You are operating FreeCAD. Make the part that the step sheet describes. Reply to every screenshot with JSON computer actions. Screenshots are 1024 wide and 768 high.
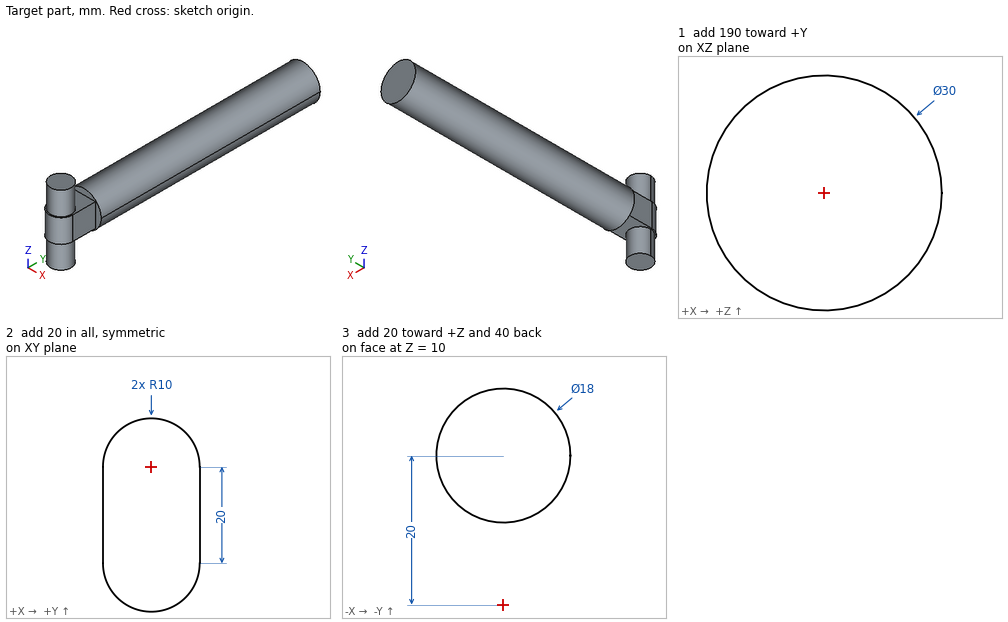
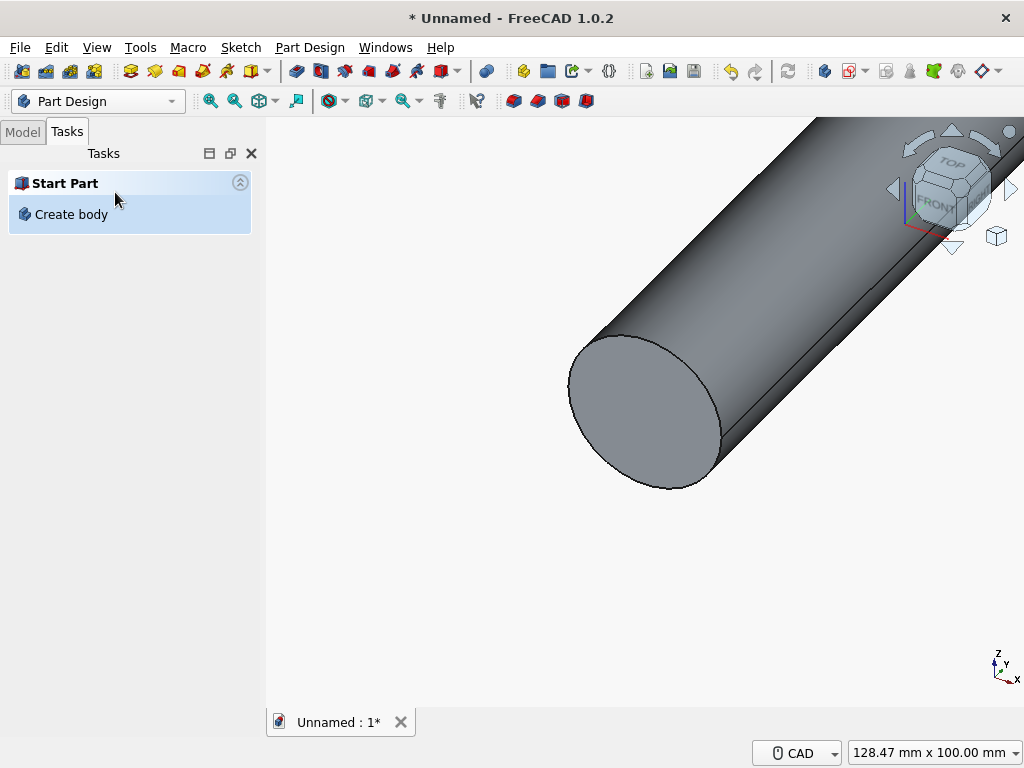
{"action": "left_click", "coordinate": [212, 102]}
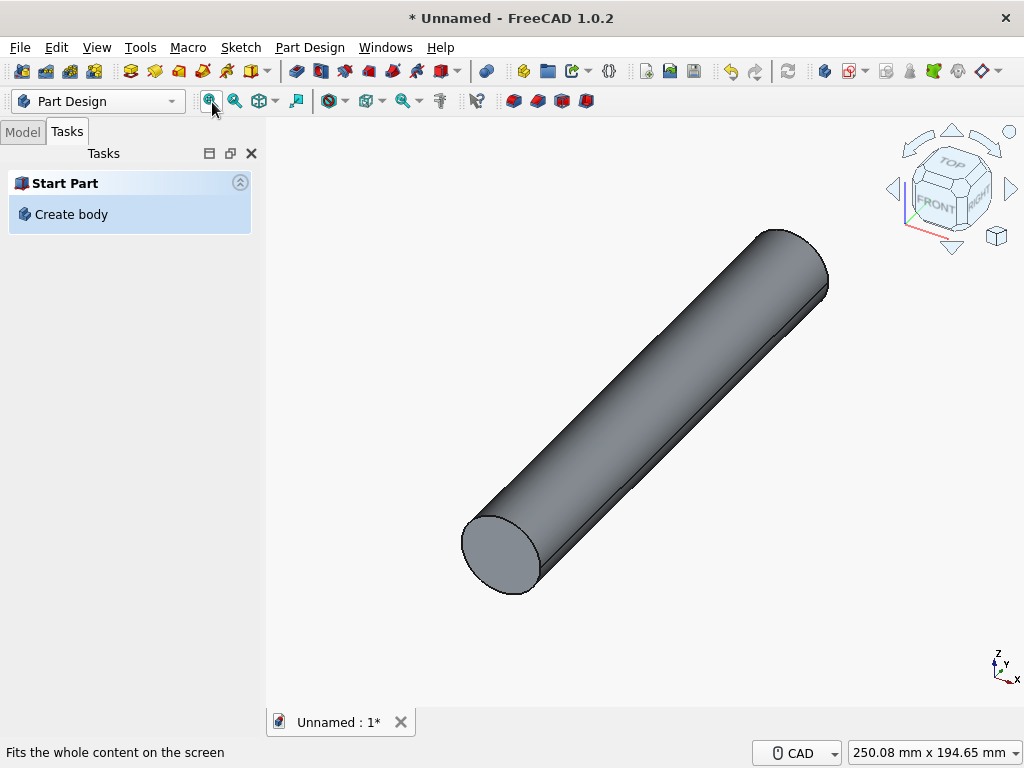
{"action": "left_click", "coordinate": [850, 72]}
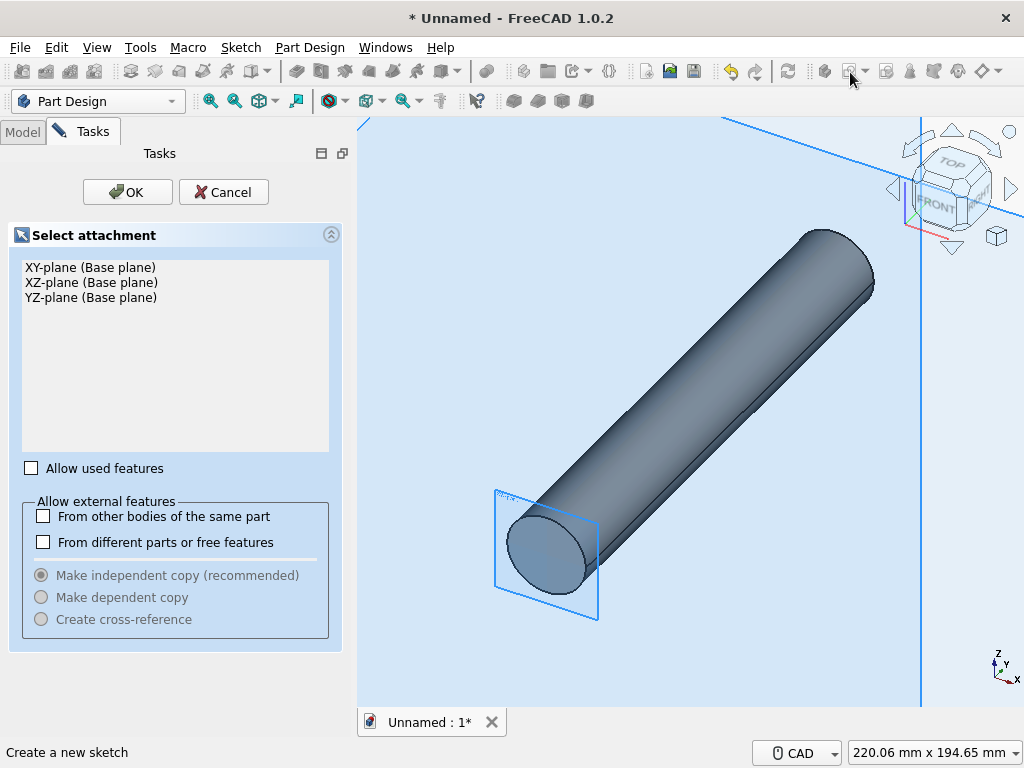
{"action": "left_click", "coordinate": [82, 268]}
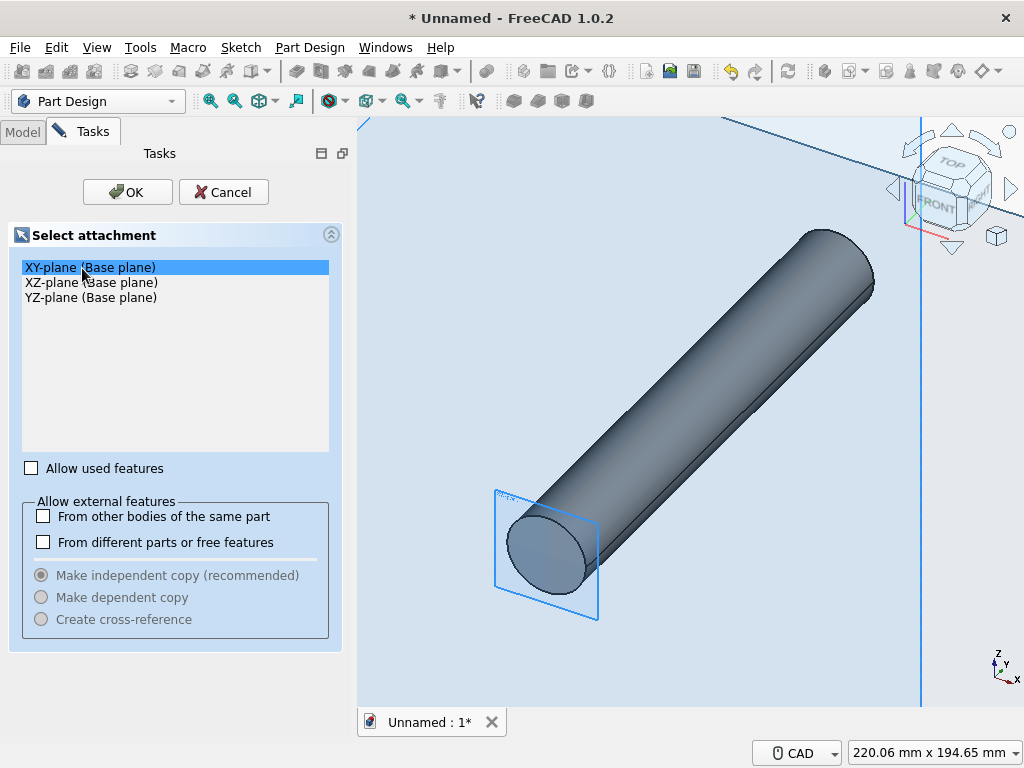
{"action": "left_click", "coordinate": [128, 192]}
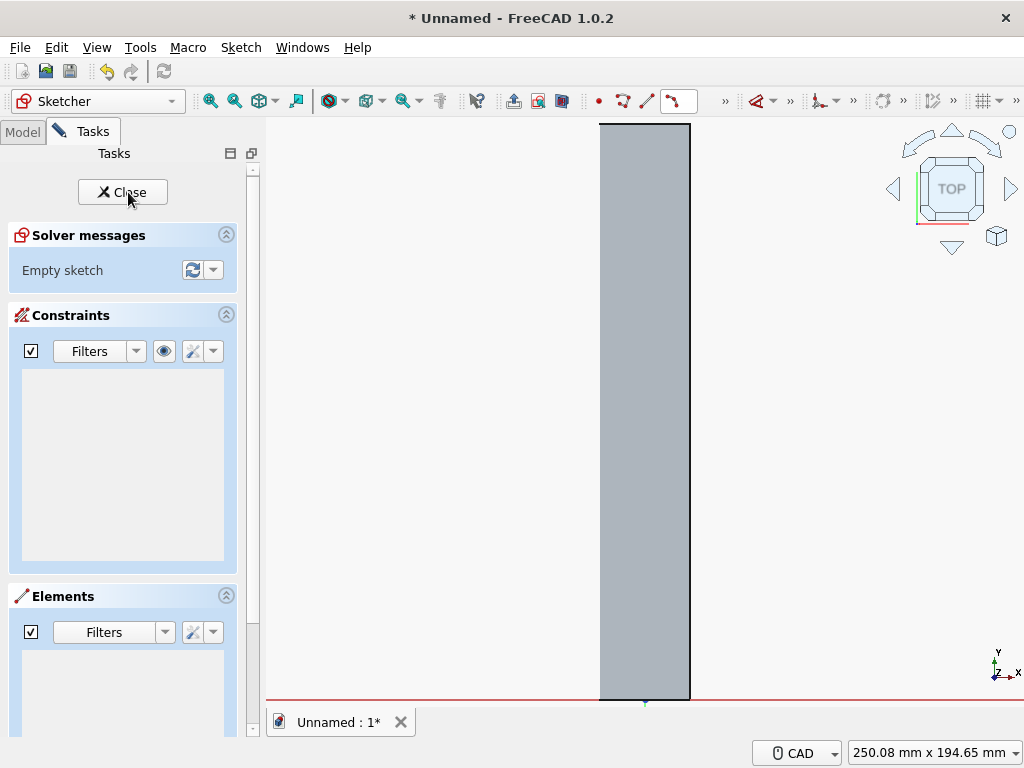
{"action": "key", "text": "q s"}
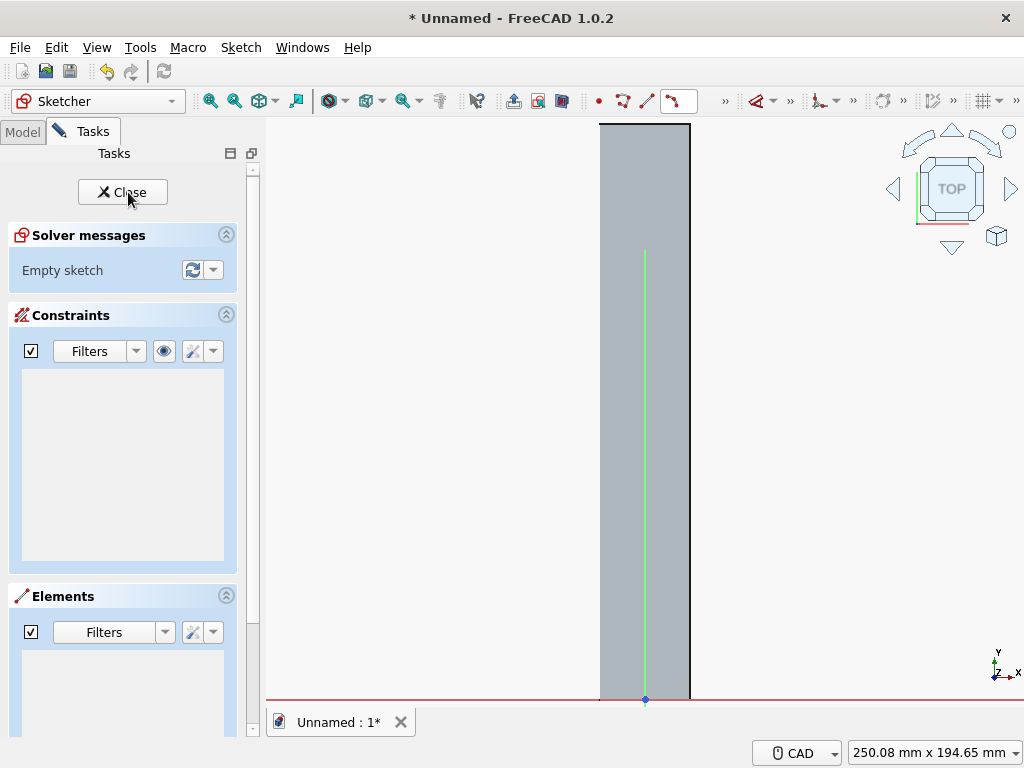
{"action": "scroll", "coordinate": [576, 412], "scroll_direction": "down", "scroll_amount": 5}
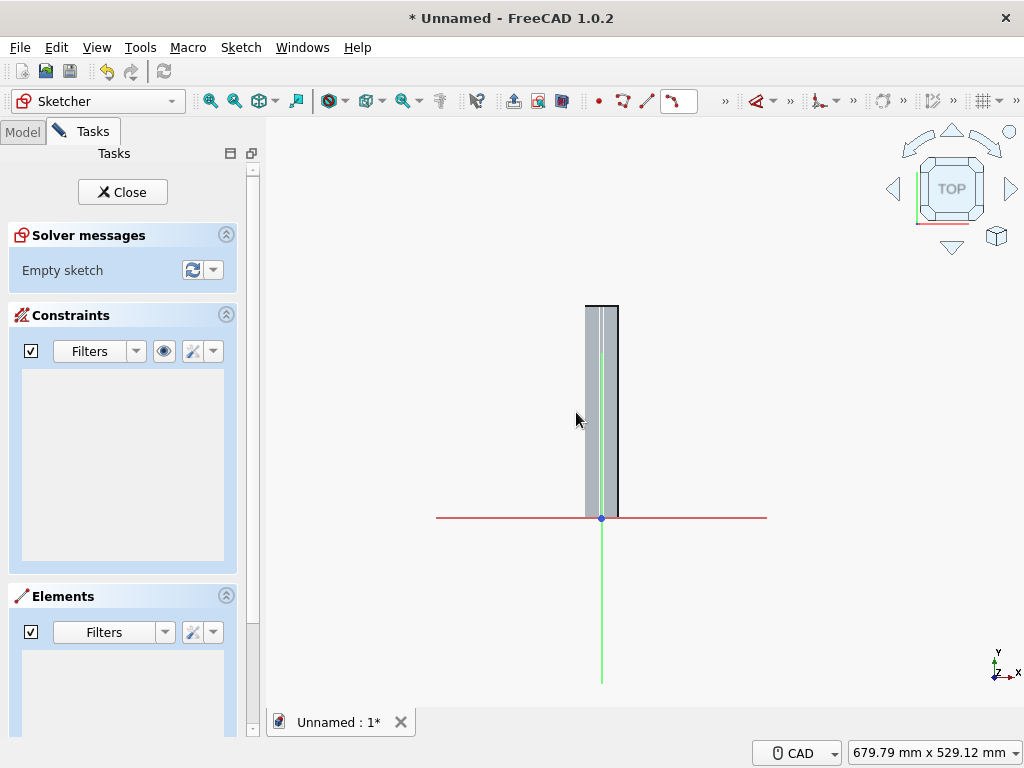
{"action": "scroll", "coordinate": [605, 544], "scroll_direction": "up", "scroll_amount": 11}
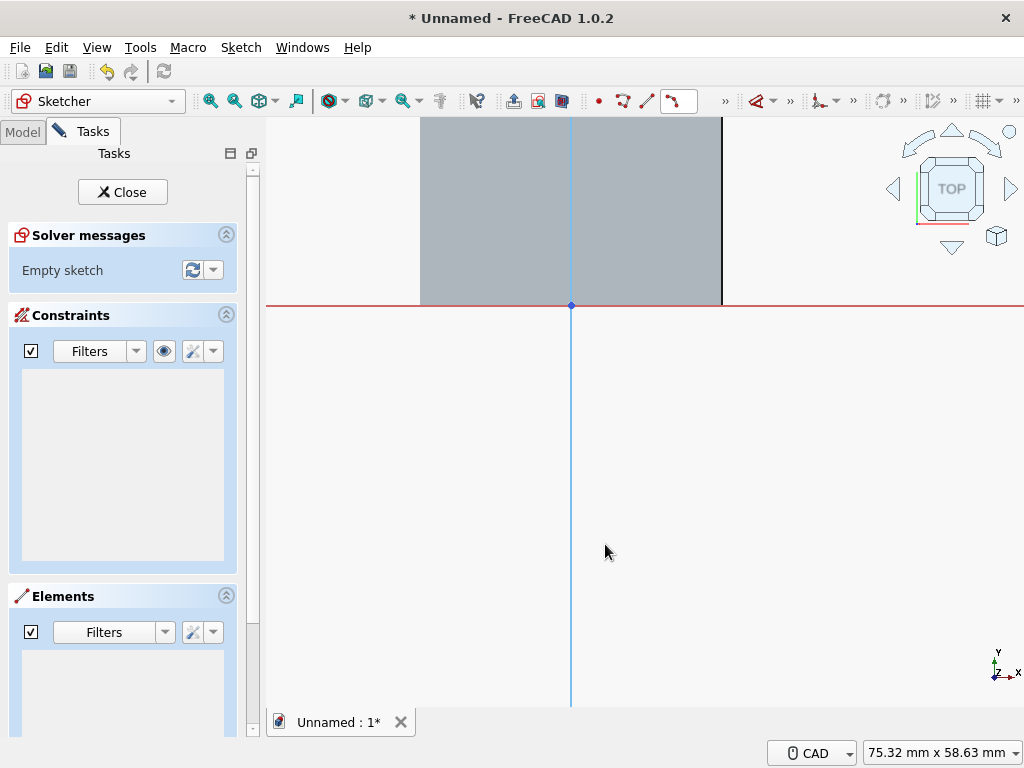
{"action": "key", "text": "g s"}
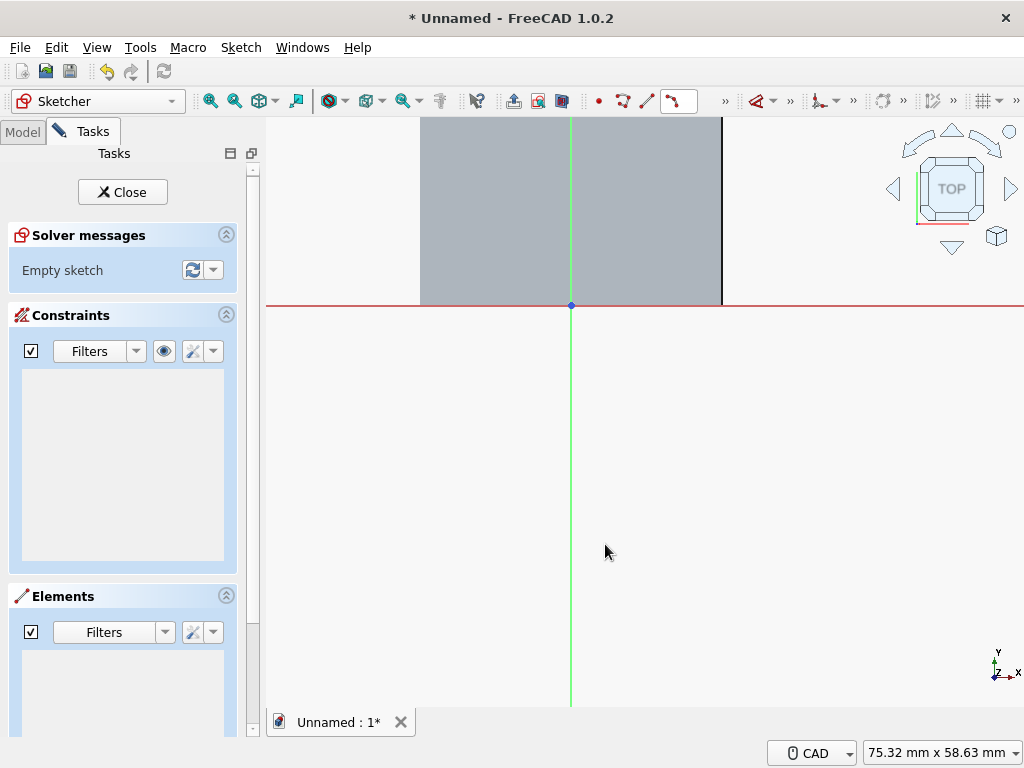
{"action": "left_click", "coordinate": [571, 306]}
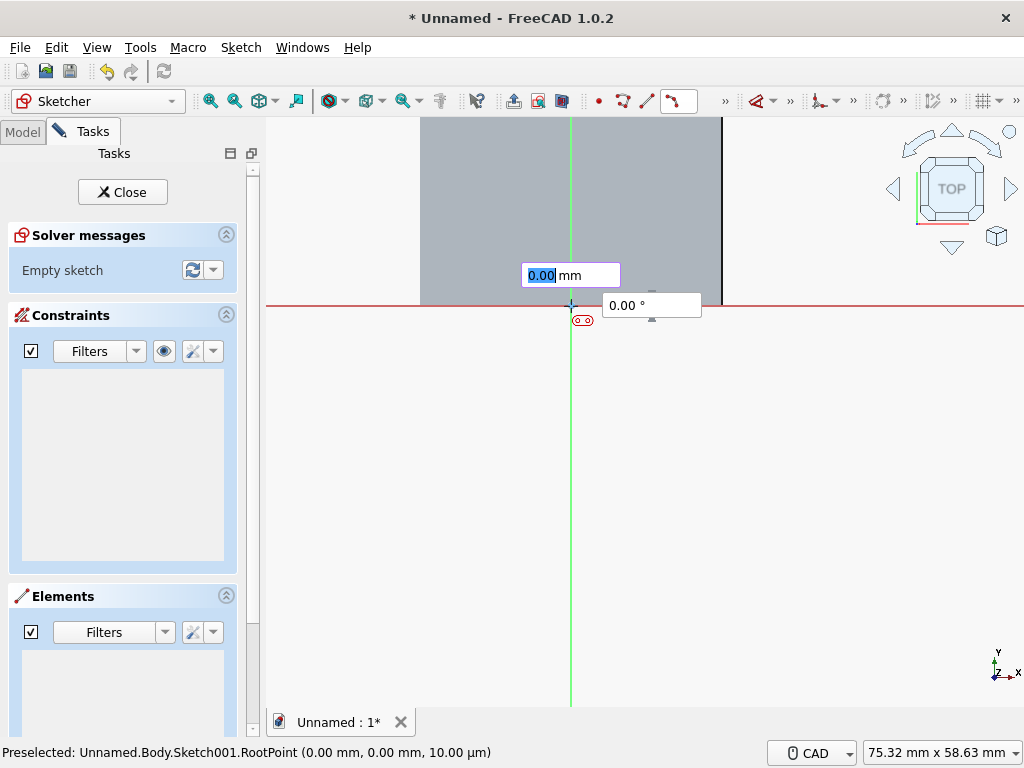
{"action": "left_click", "coordinate": [580, 507]}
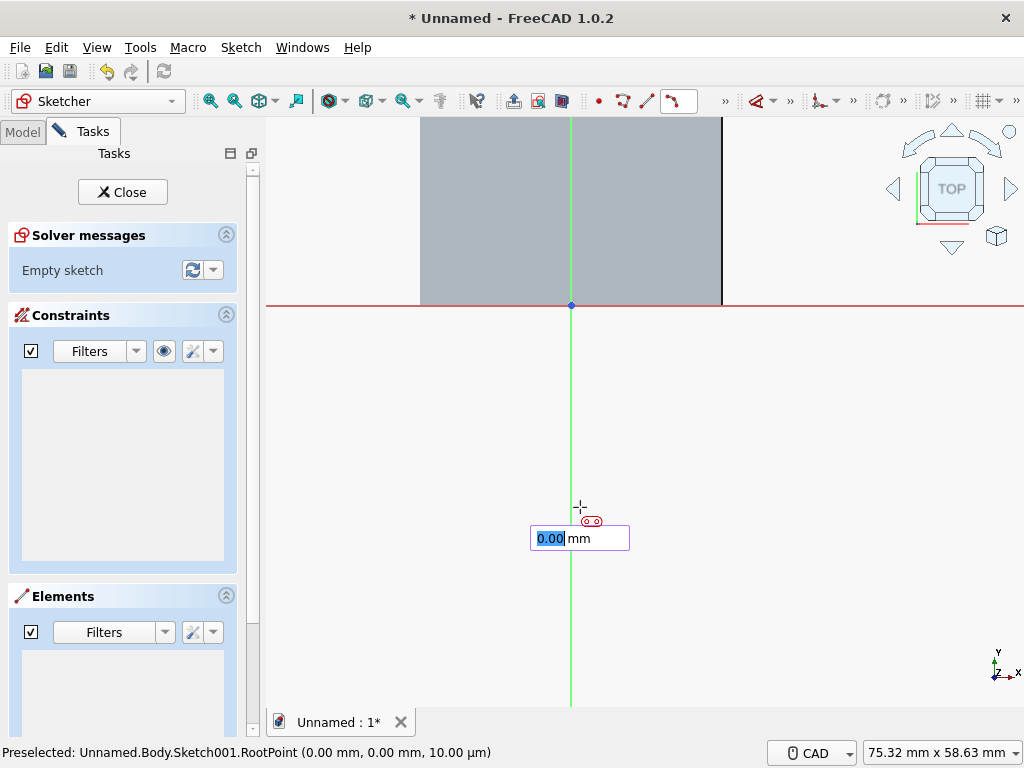
{"action": "left_click", "coordinate": [672, 406]}
{"action": "key", "text": "Escape"}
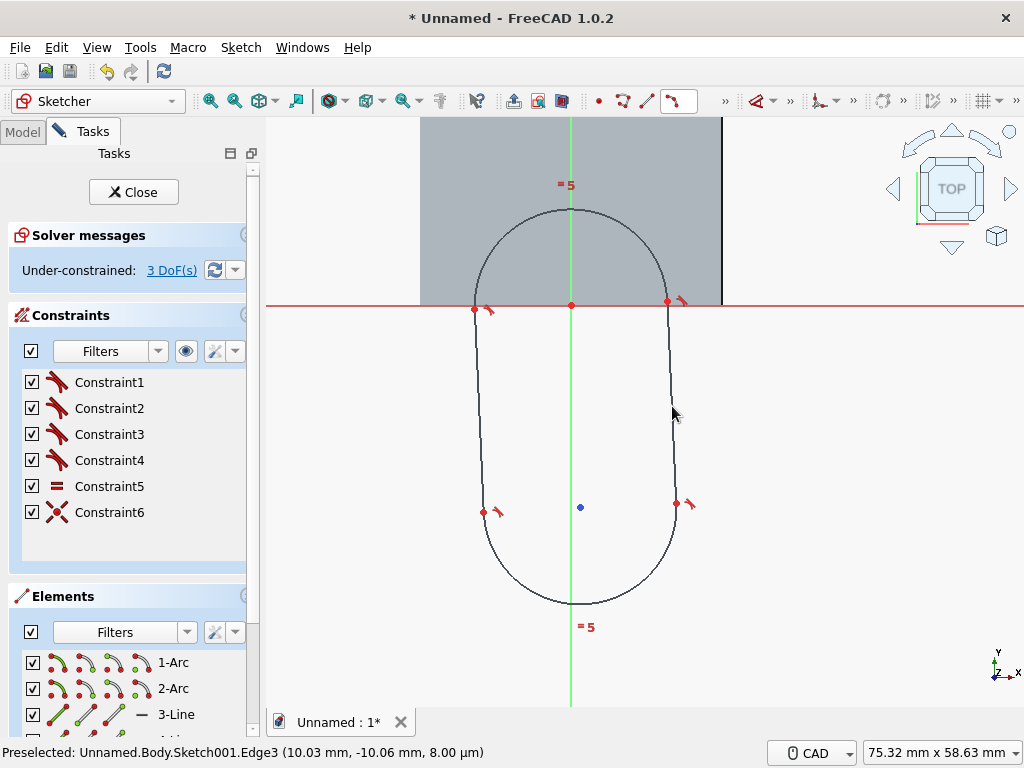
{"action": "left_click", "coordinate": [670, 362]}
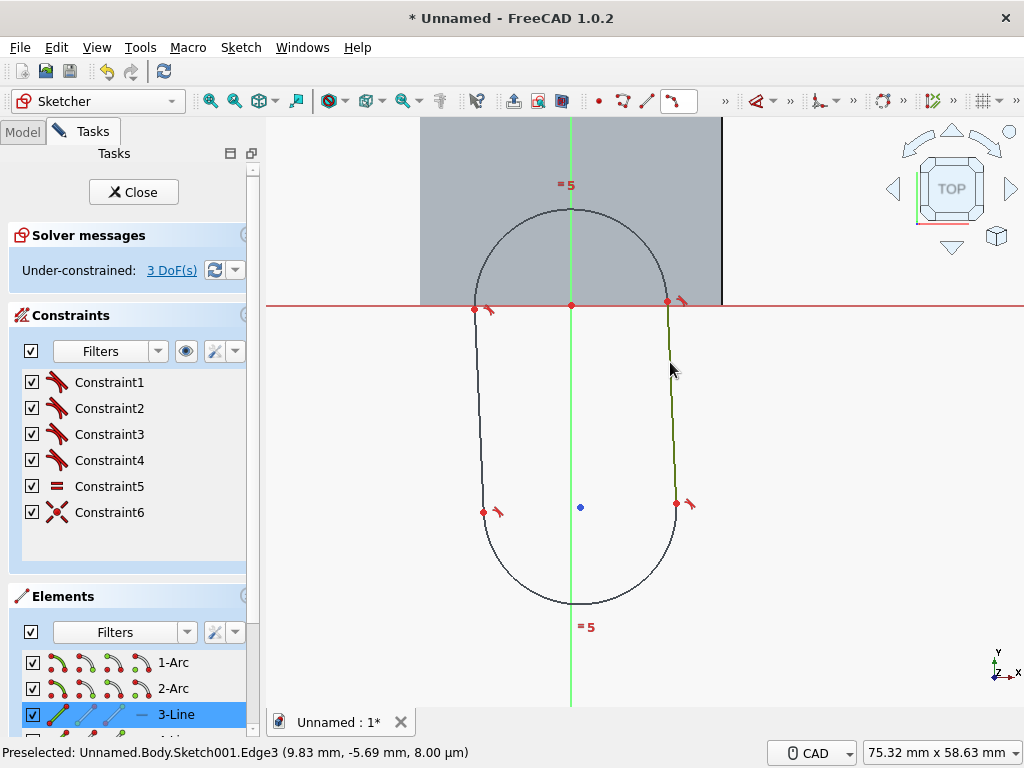
{"action": "key", "text": "v"}